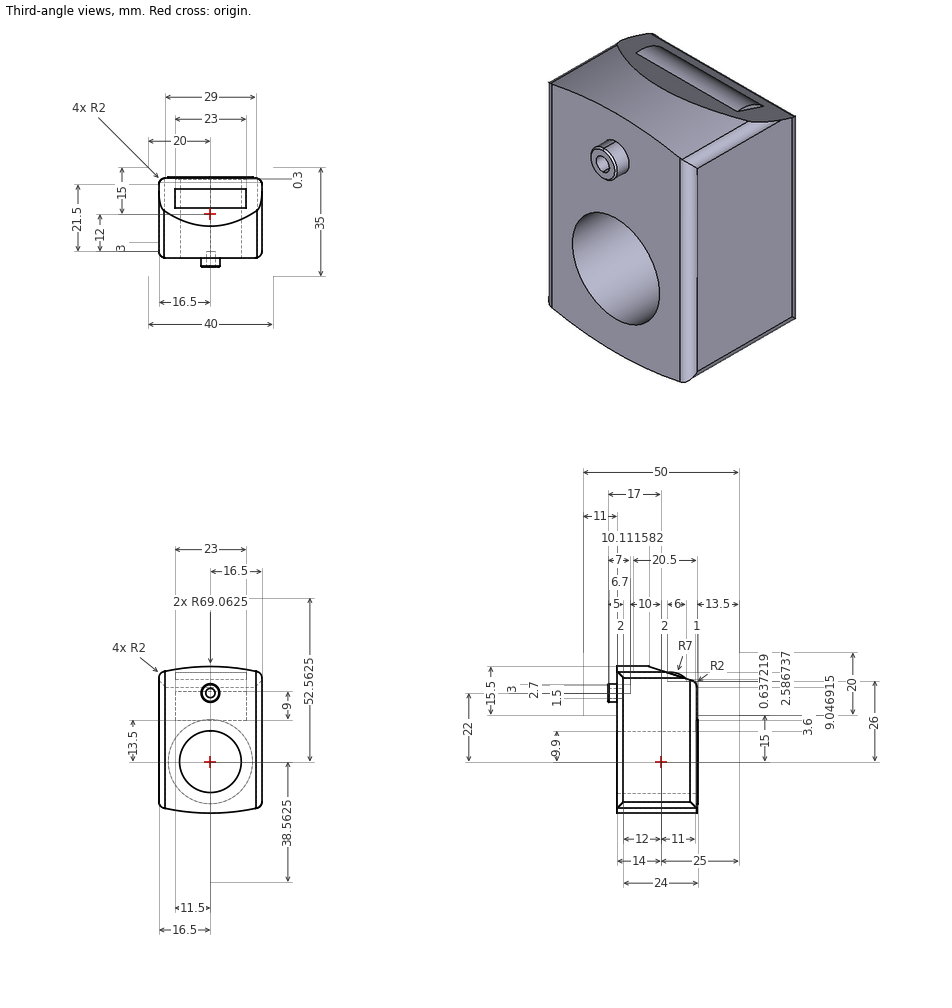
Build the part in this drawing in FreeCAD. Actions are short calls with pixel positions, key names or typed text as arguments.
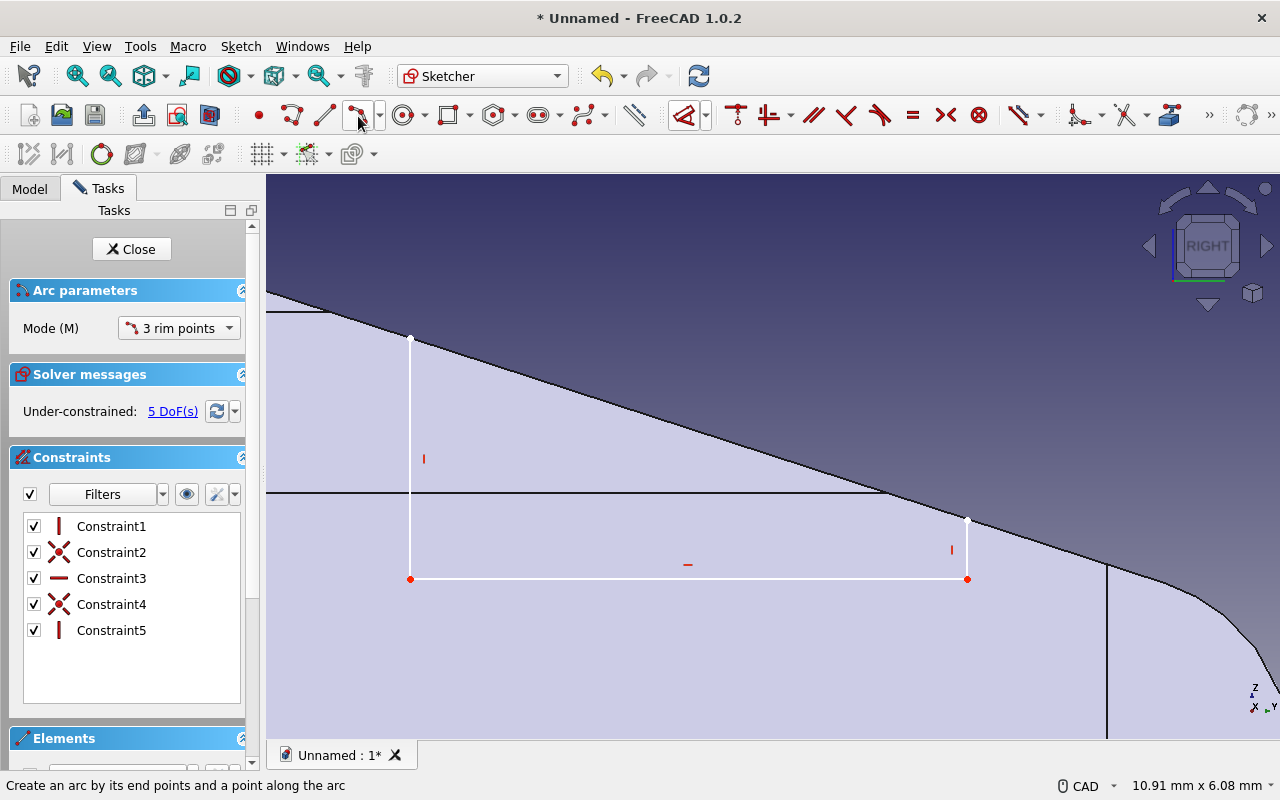
click(967, 520)
click(410, 339)
click(710, 362)
key(Escape)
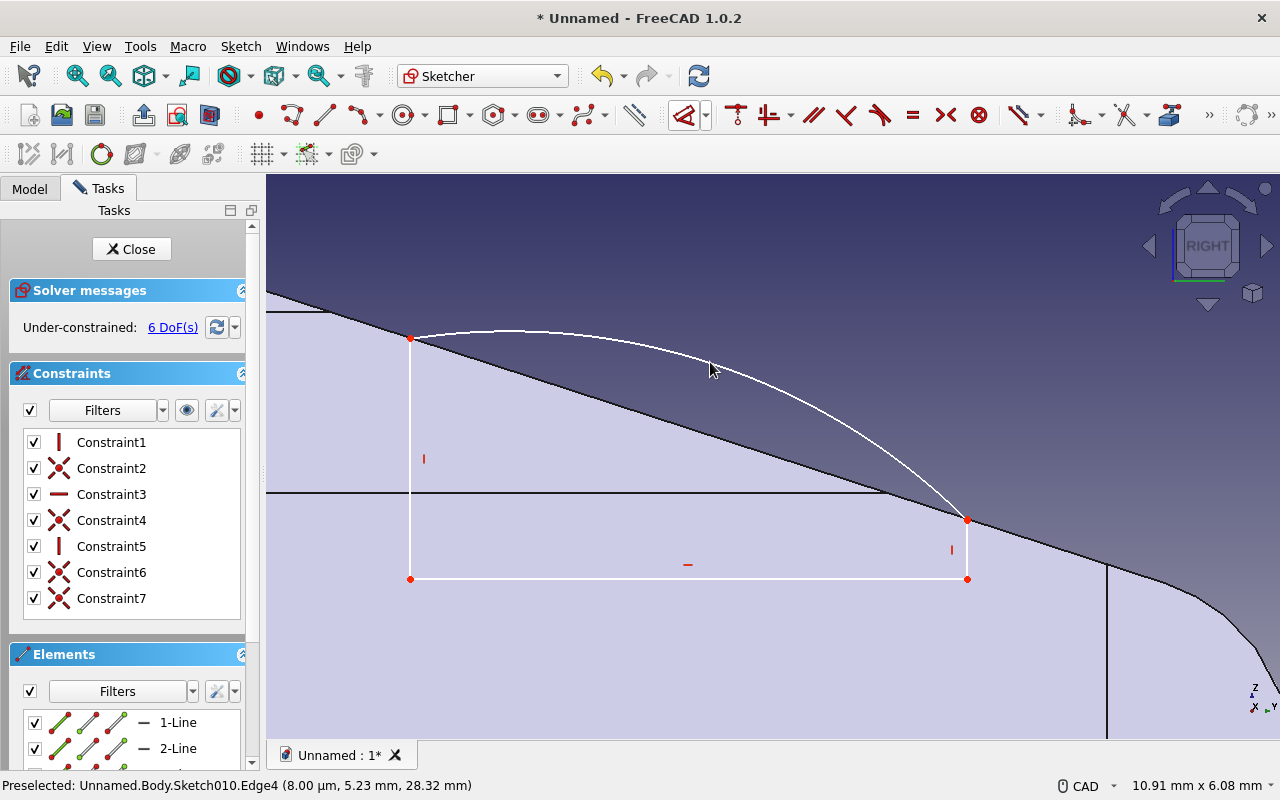
click(821, 411)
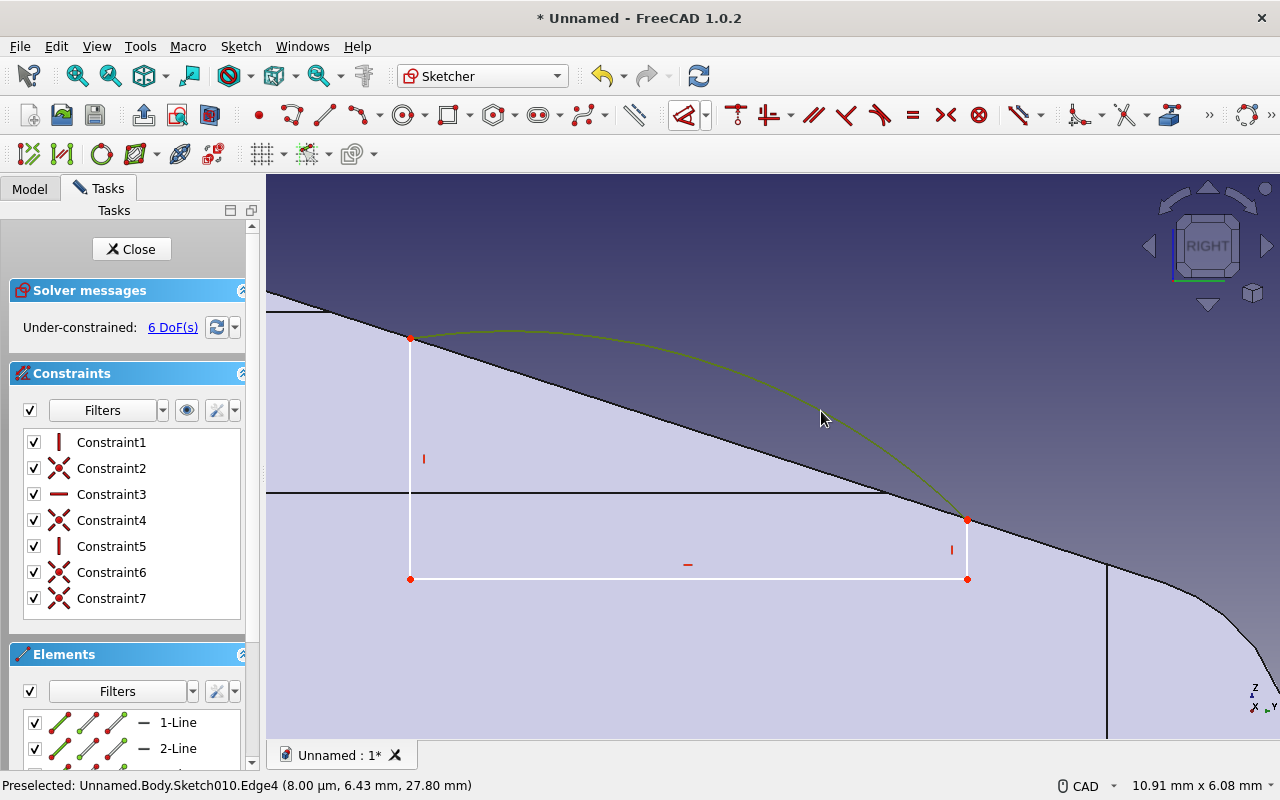
key(k)
key(r)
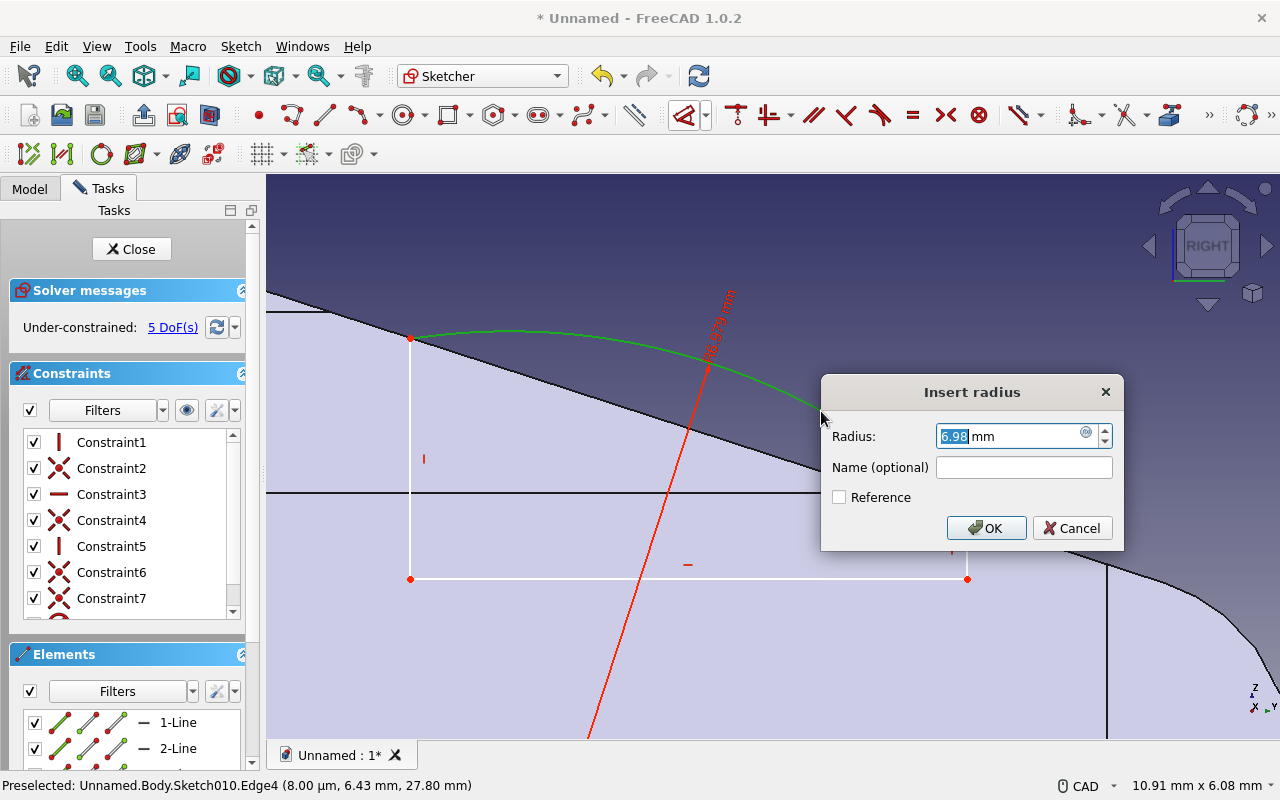
text(7)
key(Return)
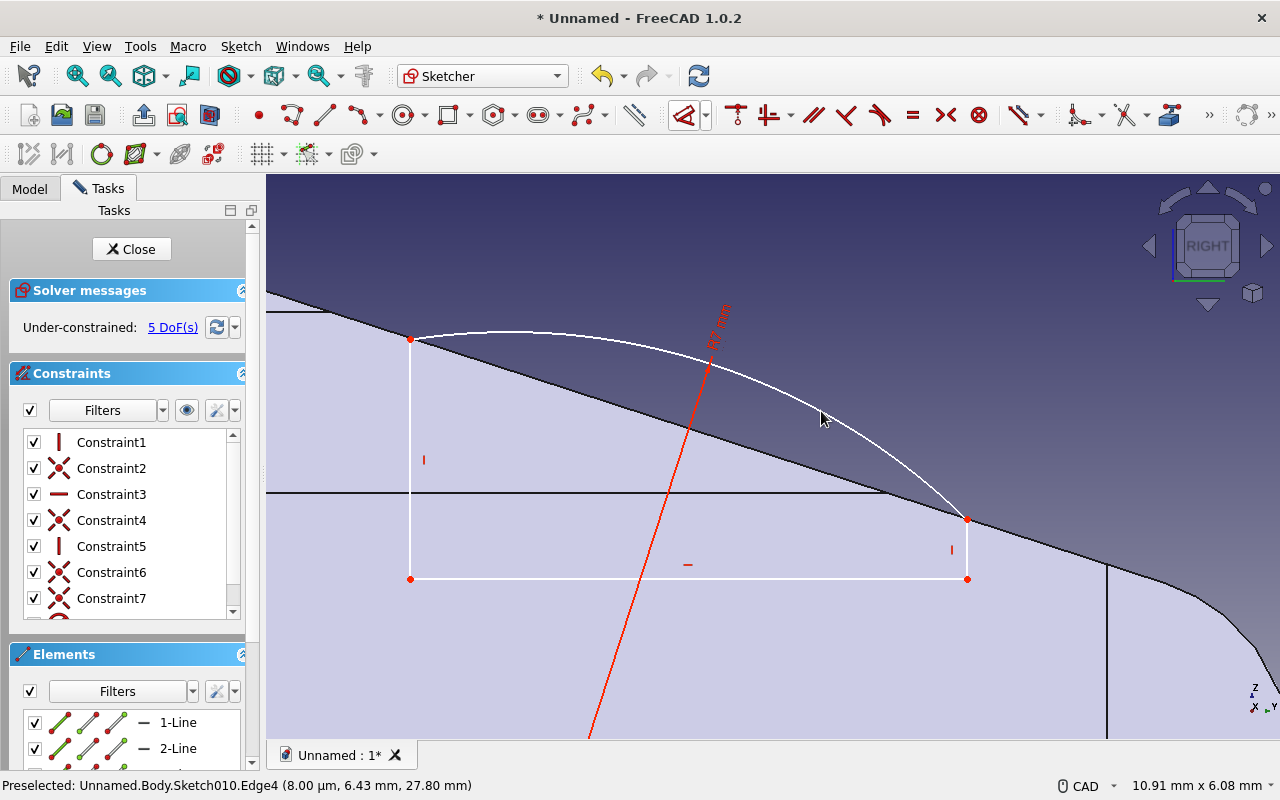
click(577, 579)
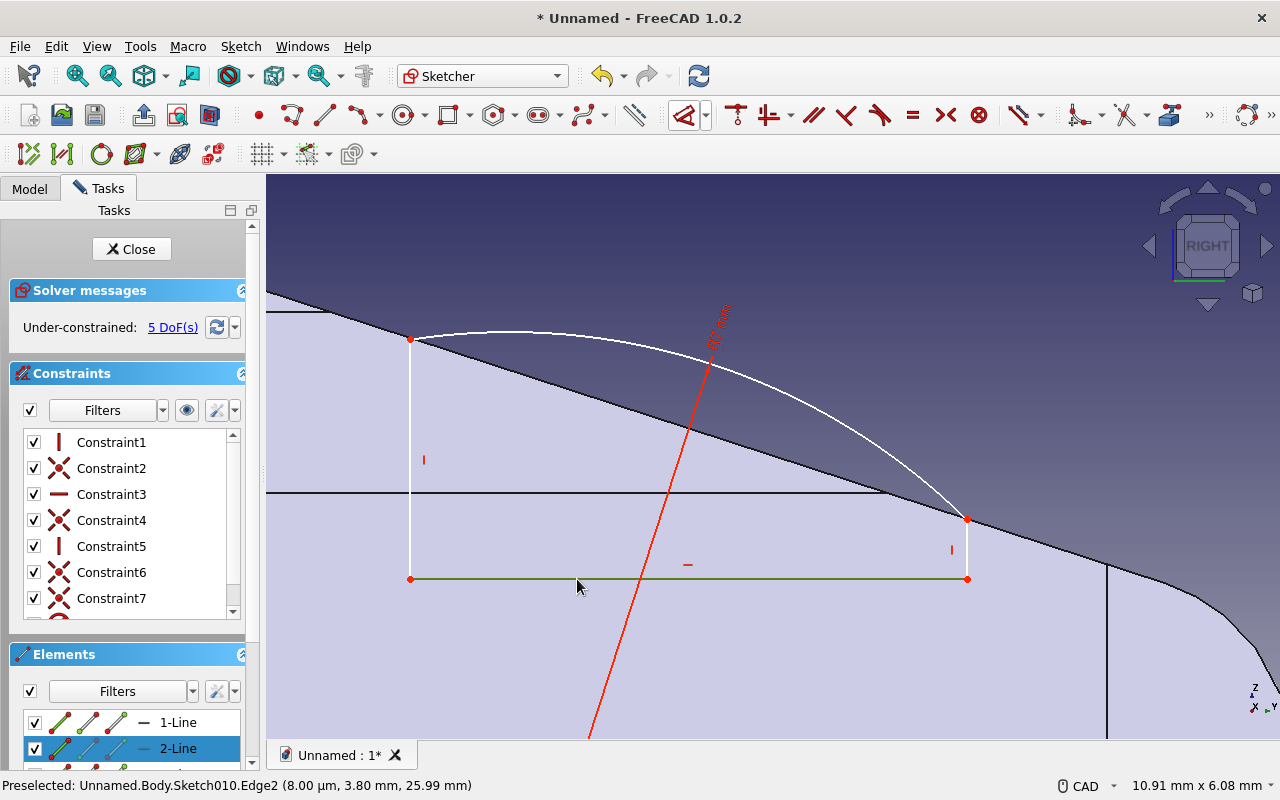
click(706, 116)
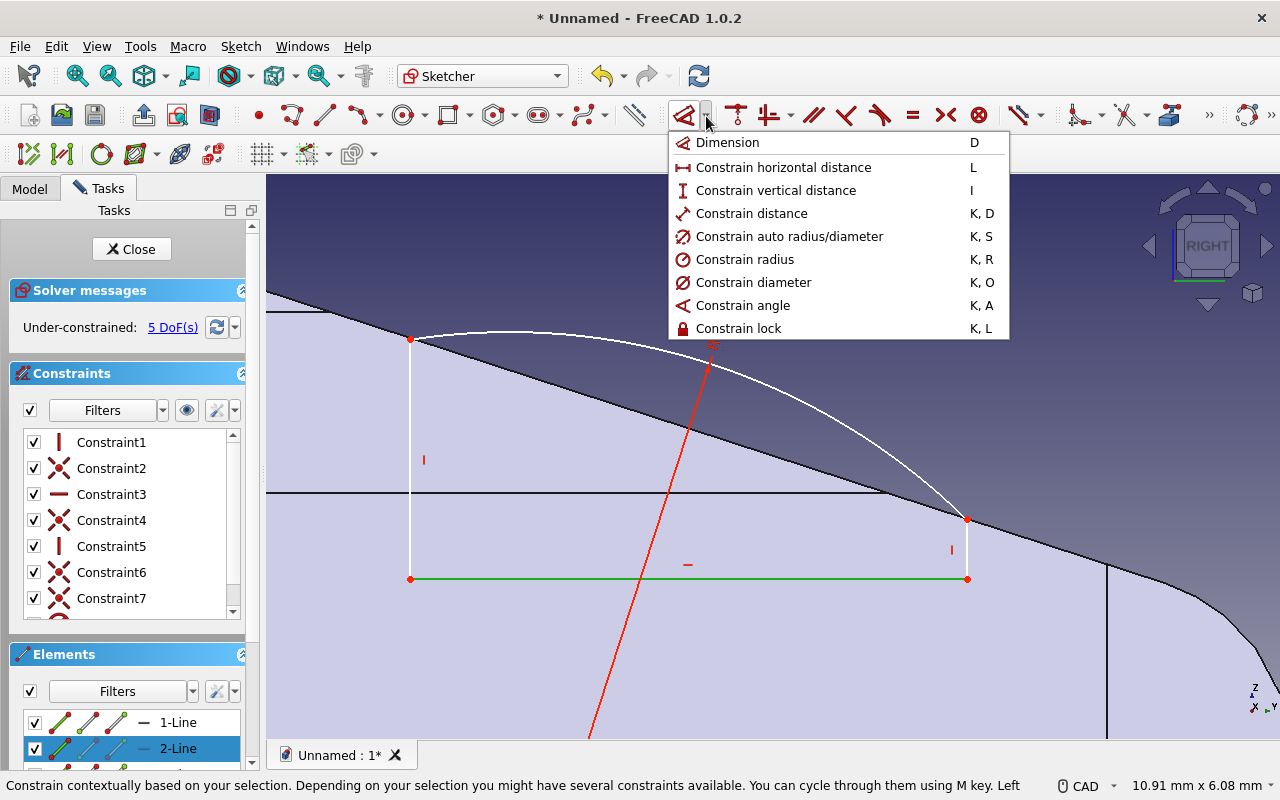
click(839, 168)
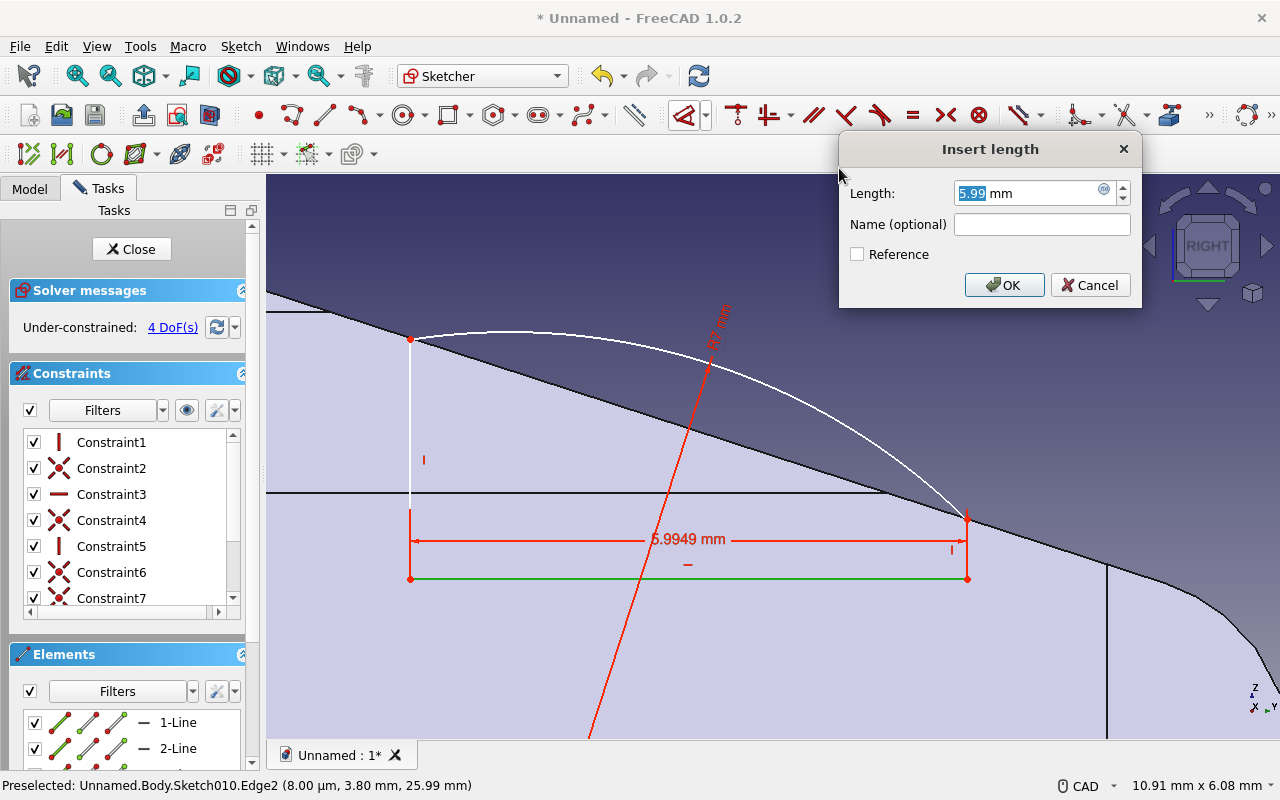
text(6)
key(Return)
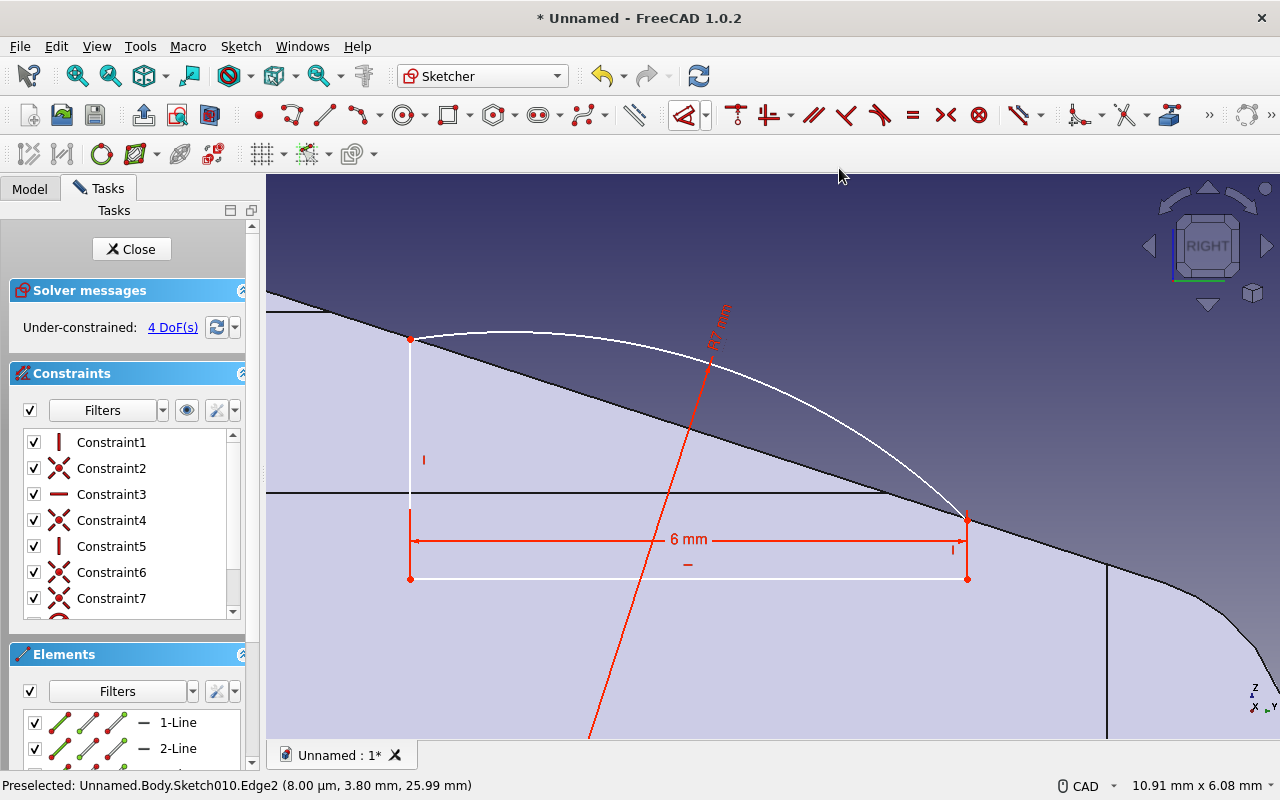
click(410, 340)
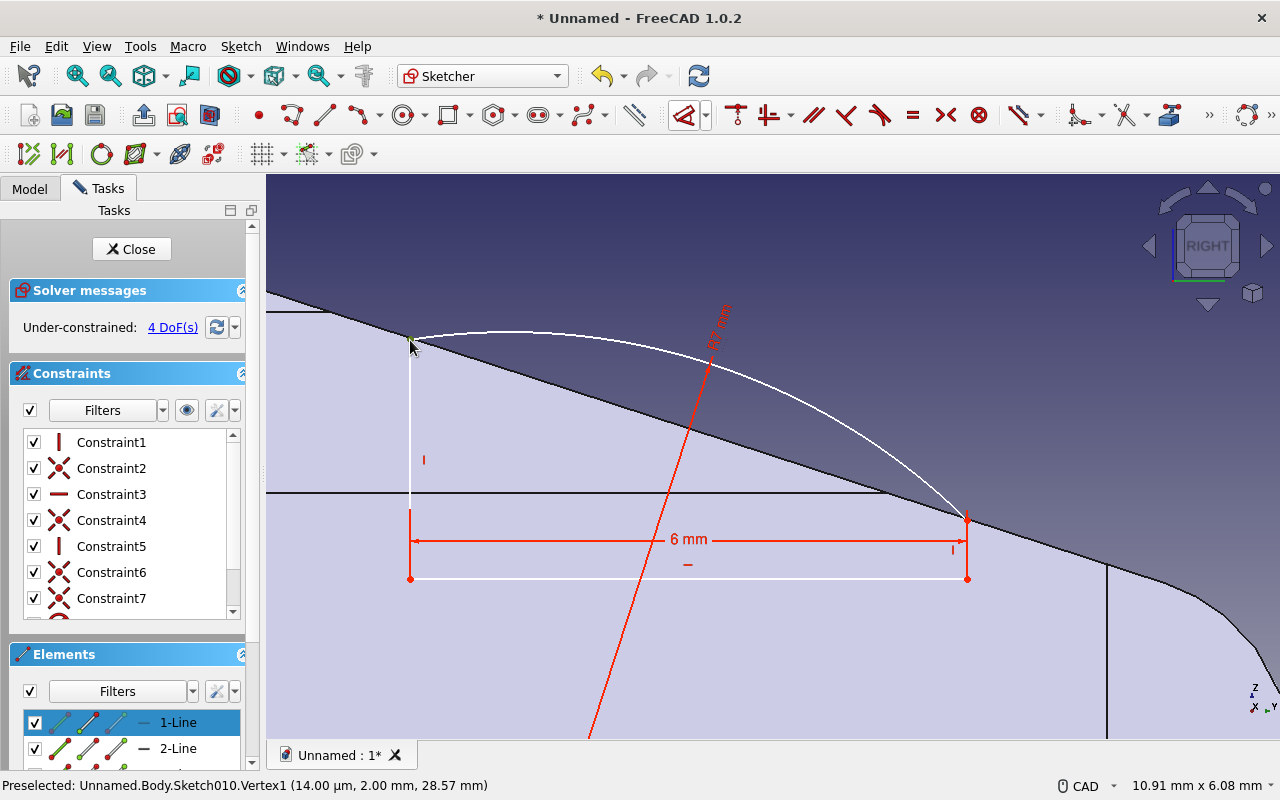
click(706, 116)